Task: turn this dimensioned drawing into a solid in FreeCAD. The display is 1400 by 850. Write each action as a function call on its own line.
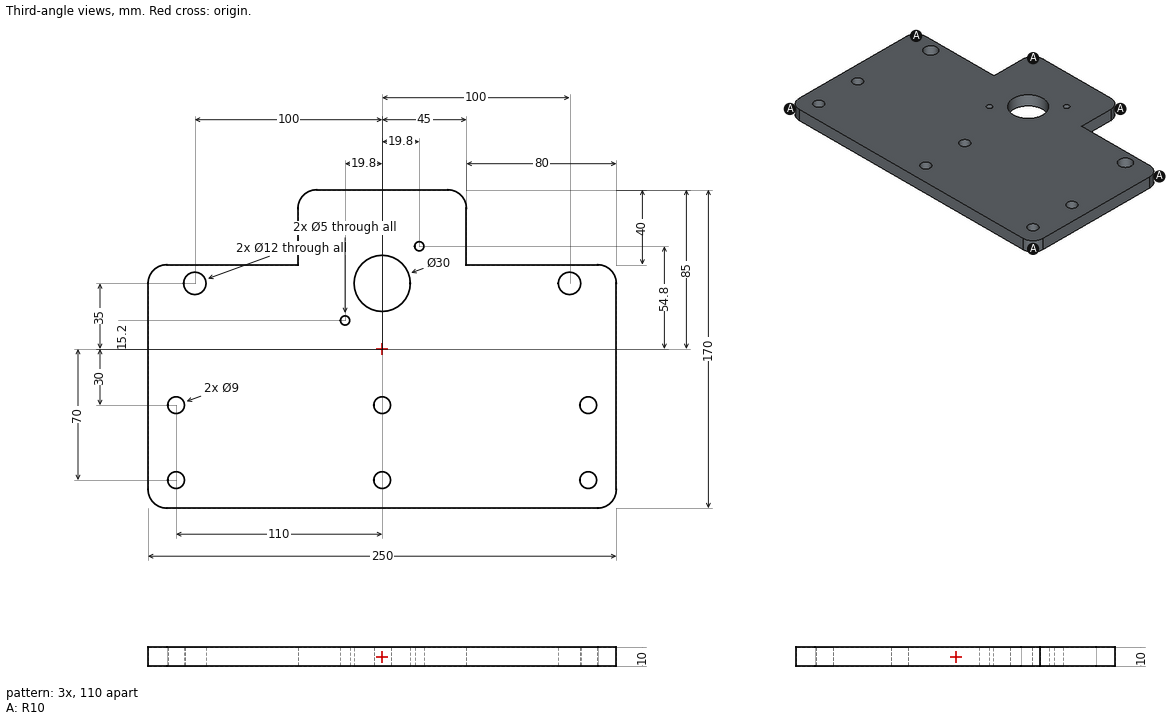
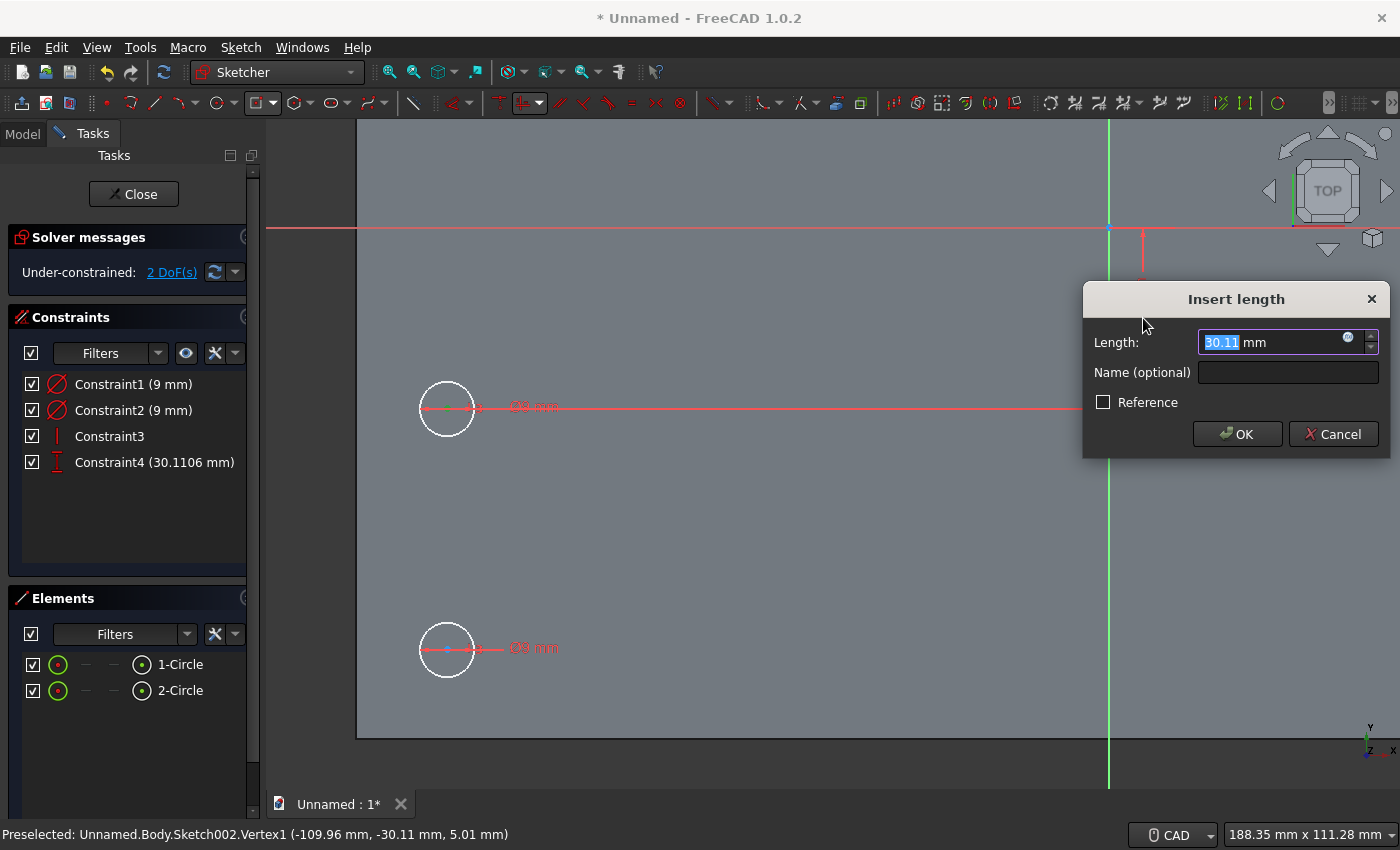
text(30)
key(Return)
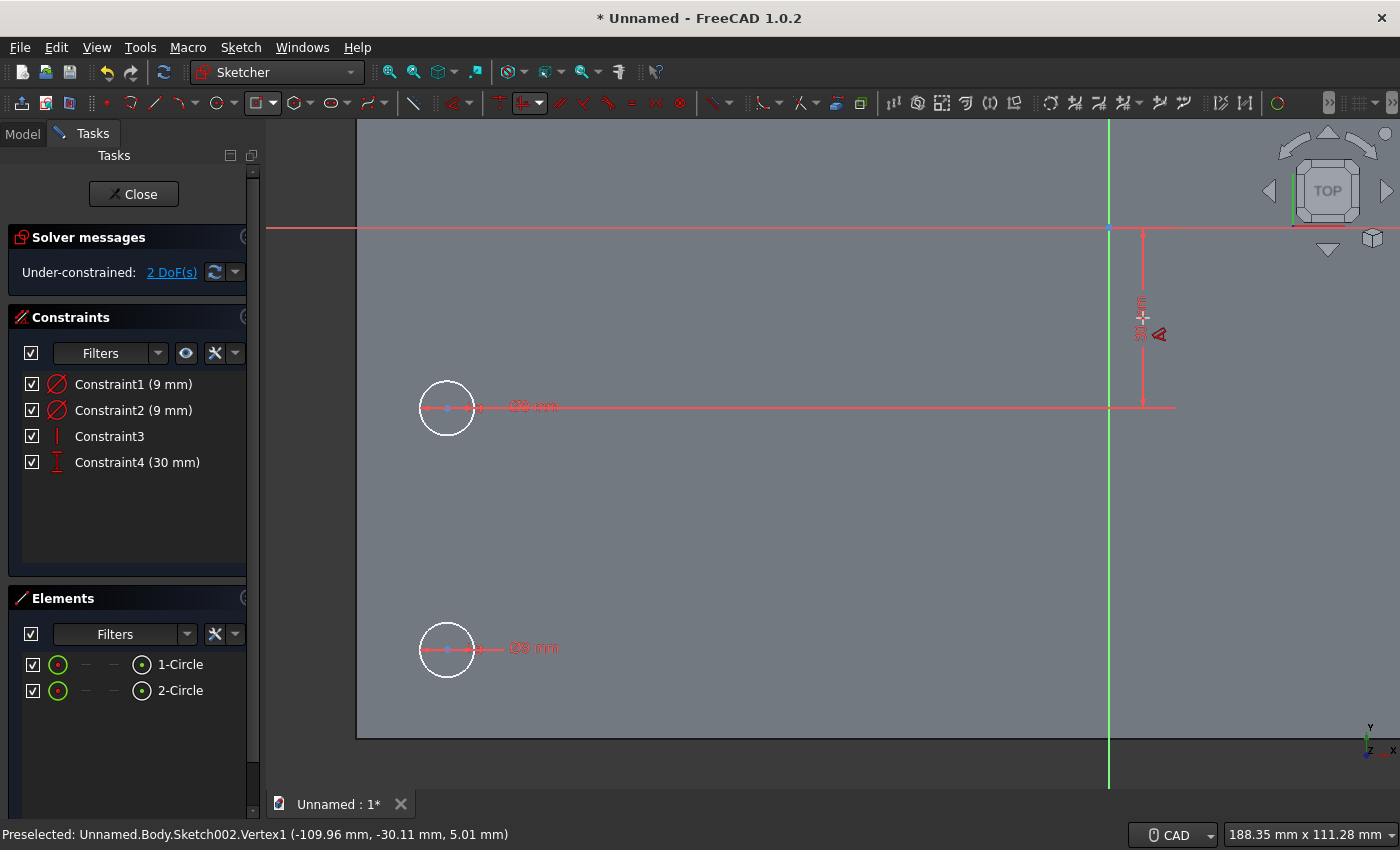
click(447, 650)
click(1143, 439)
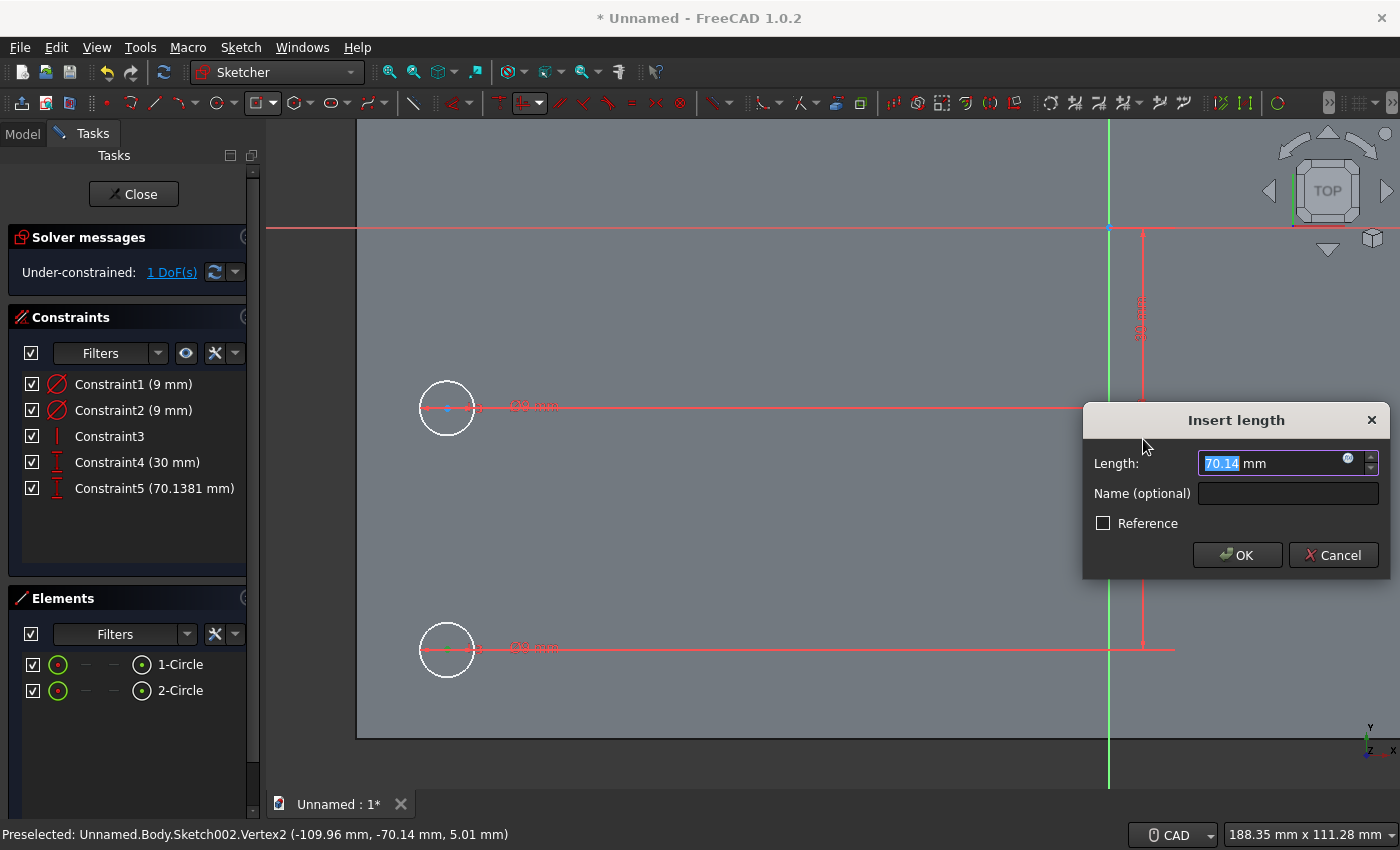
text(70)
key(Return)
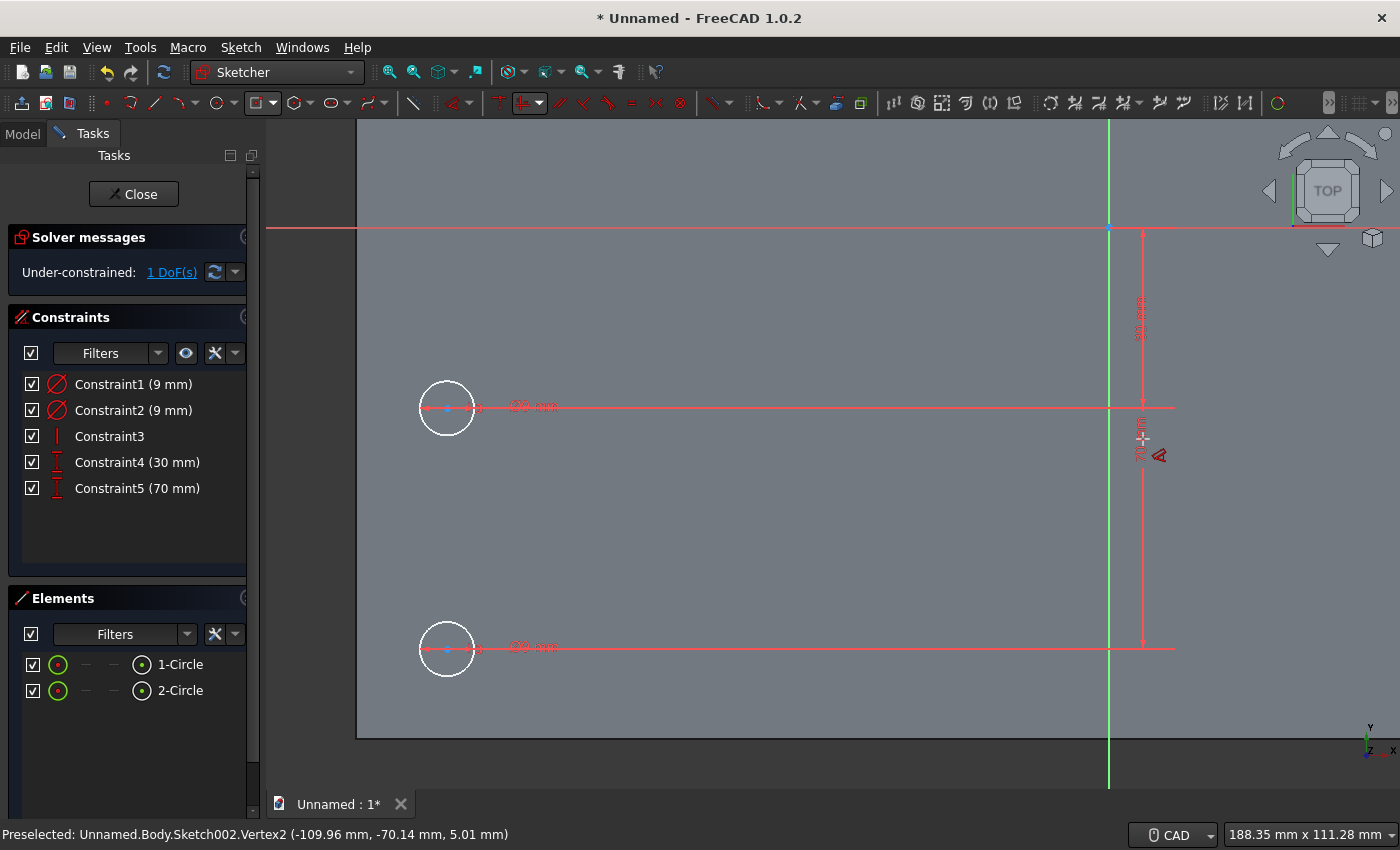
click(447, 408)
click(778, 194)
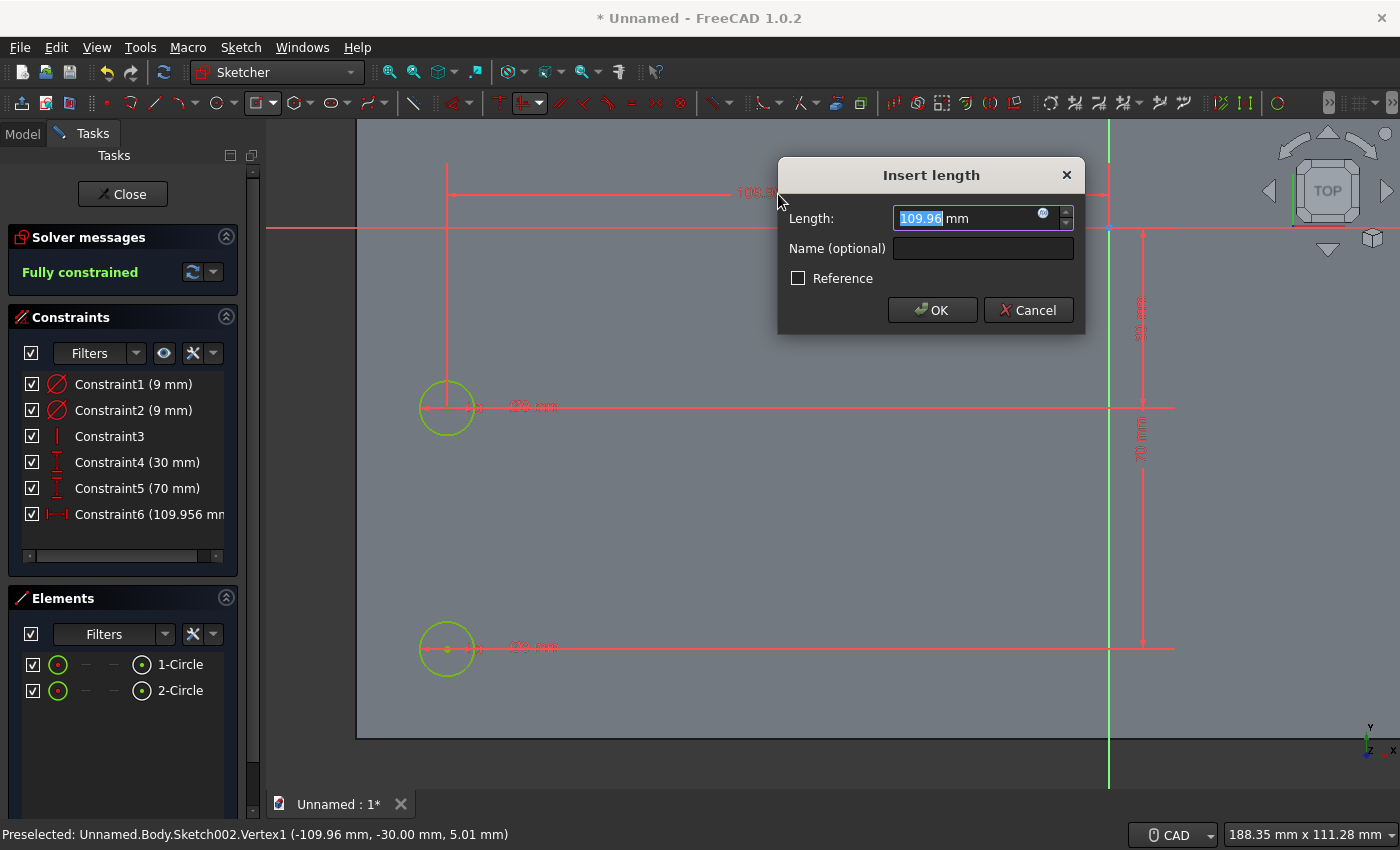
text(110)
key(Return)
key(Escape)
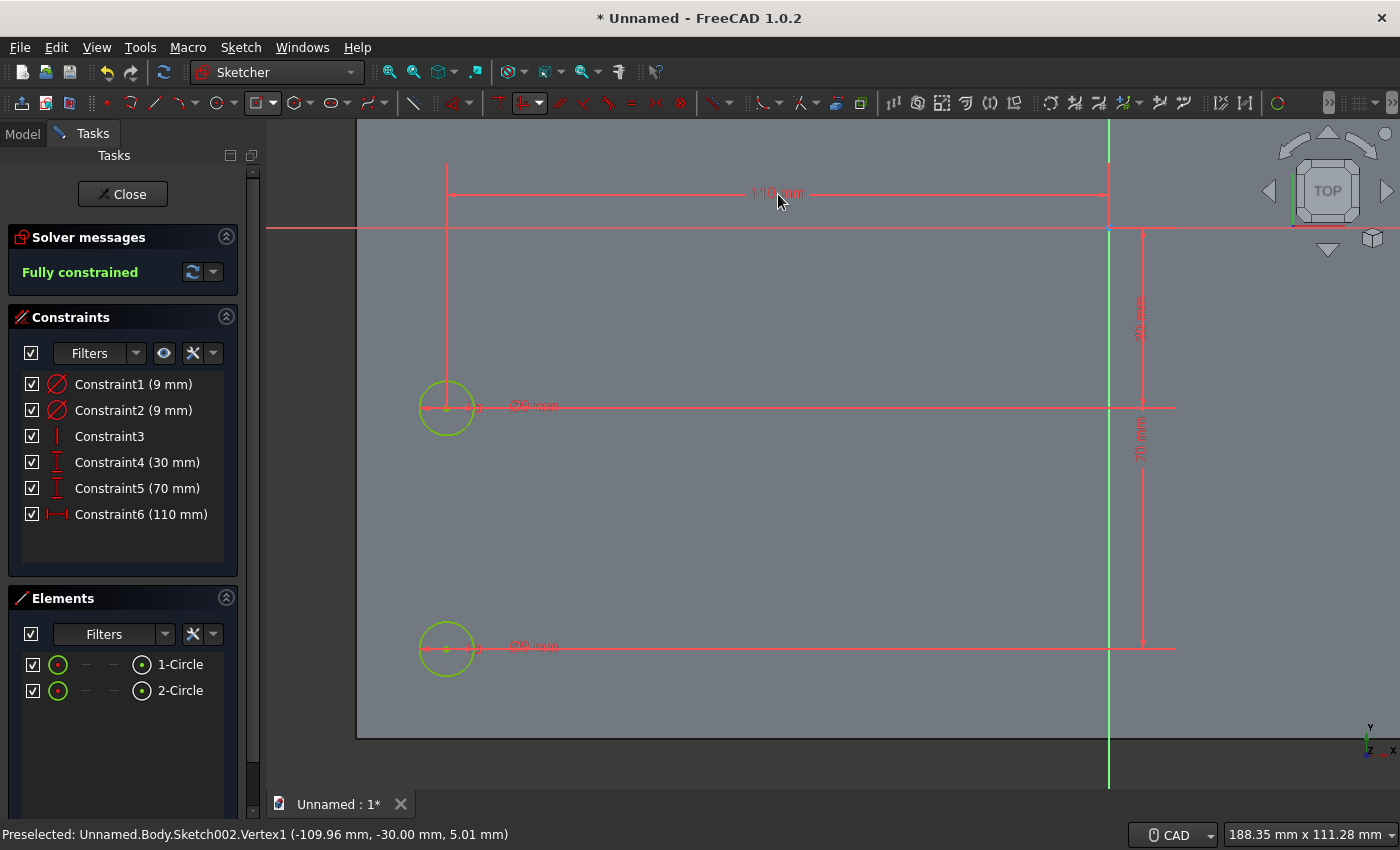
click(123, 194)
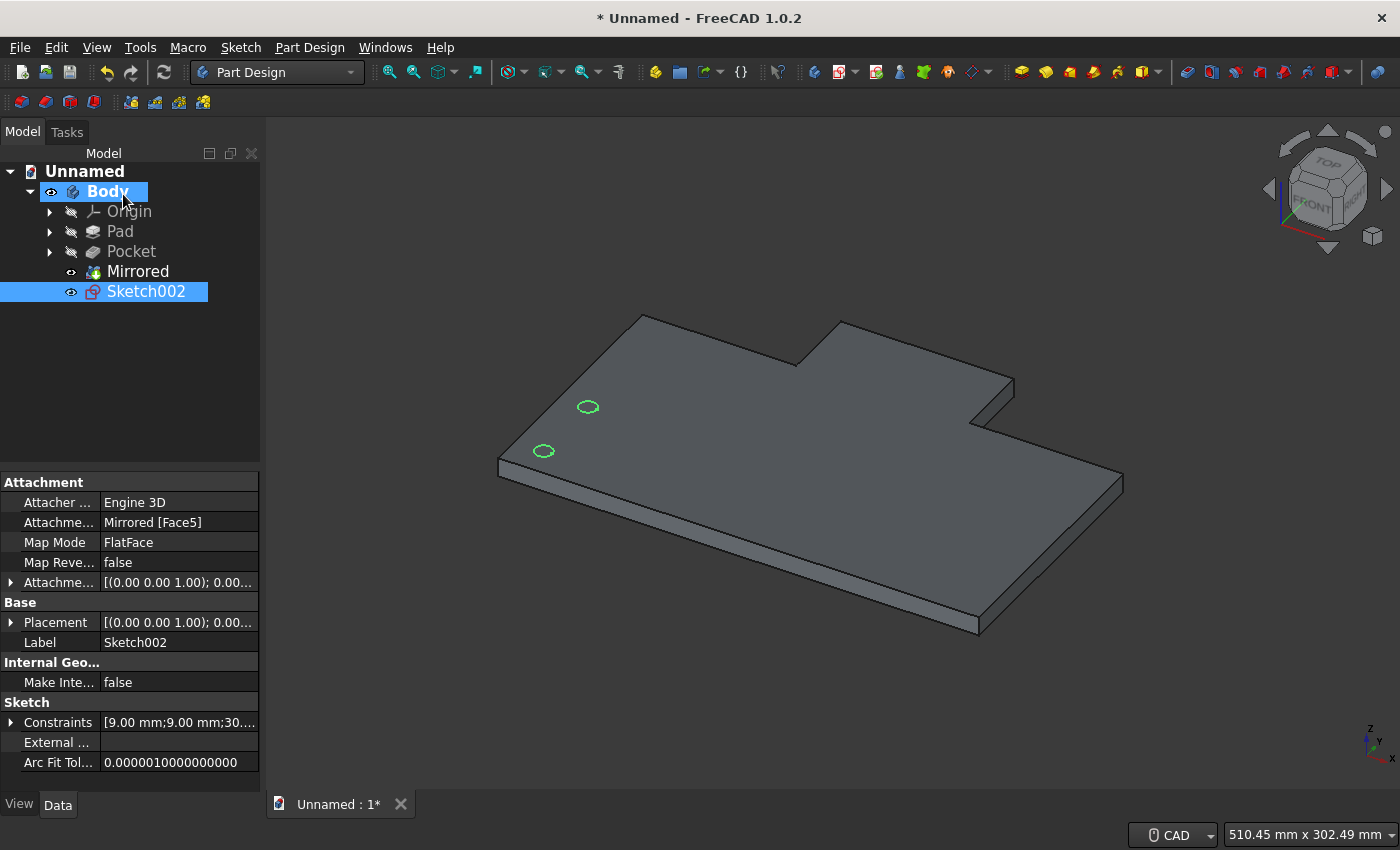
click(1188, 72)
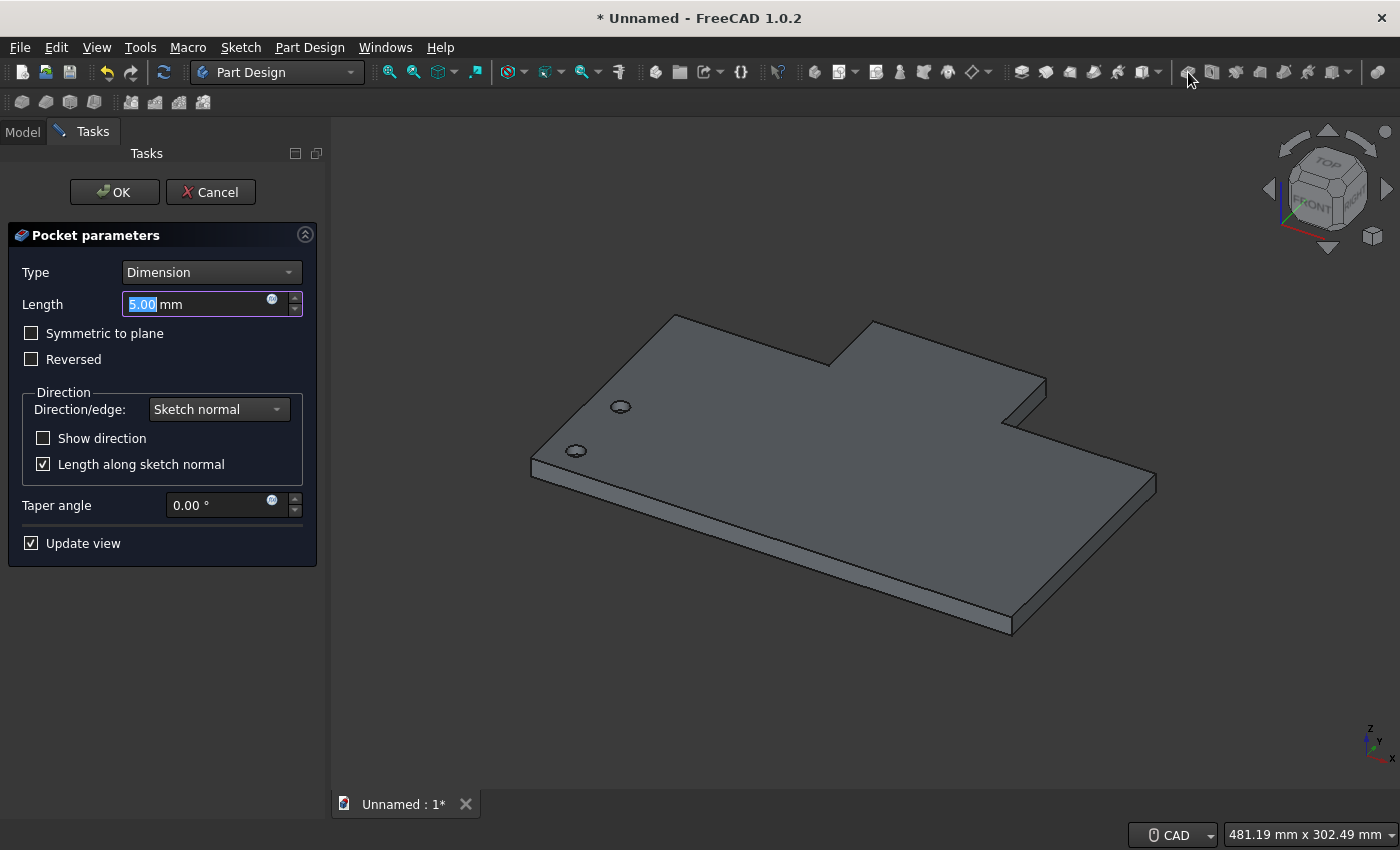
click(212, 272)